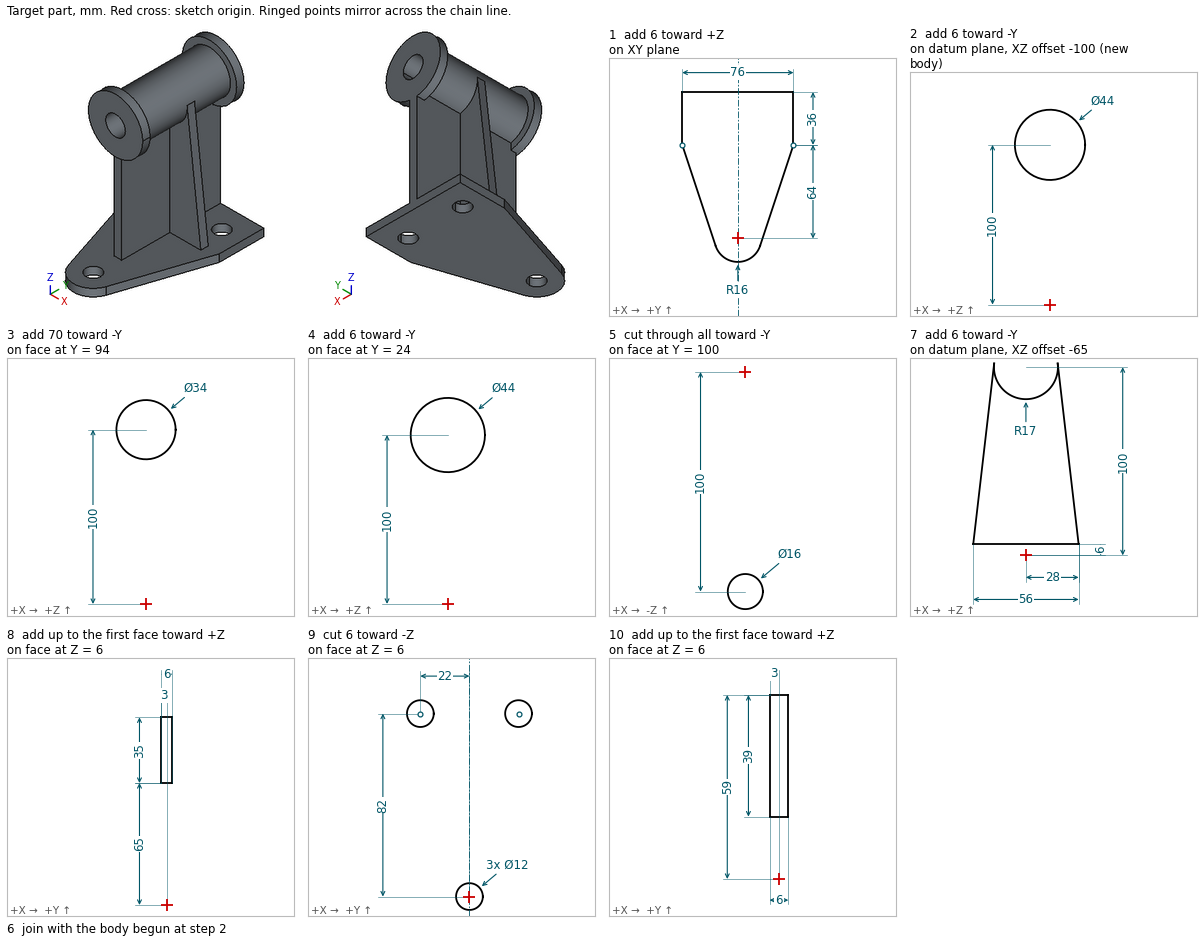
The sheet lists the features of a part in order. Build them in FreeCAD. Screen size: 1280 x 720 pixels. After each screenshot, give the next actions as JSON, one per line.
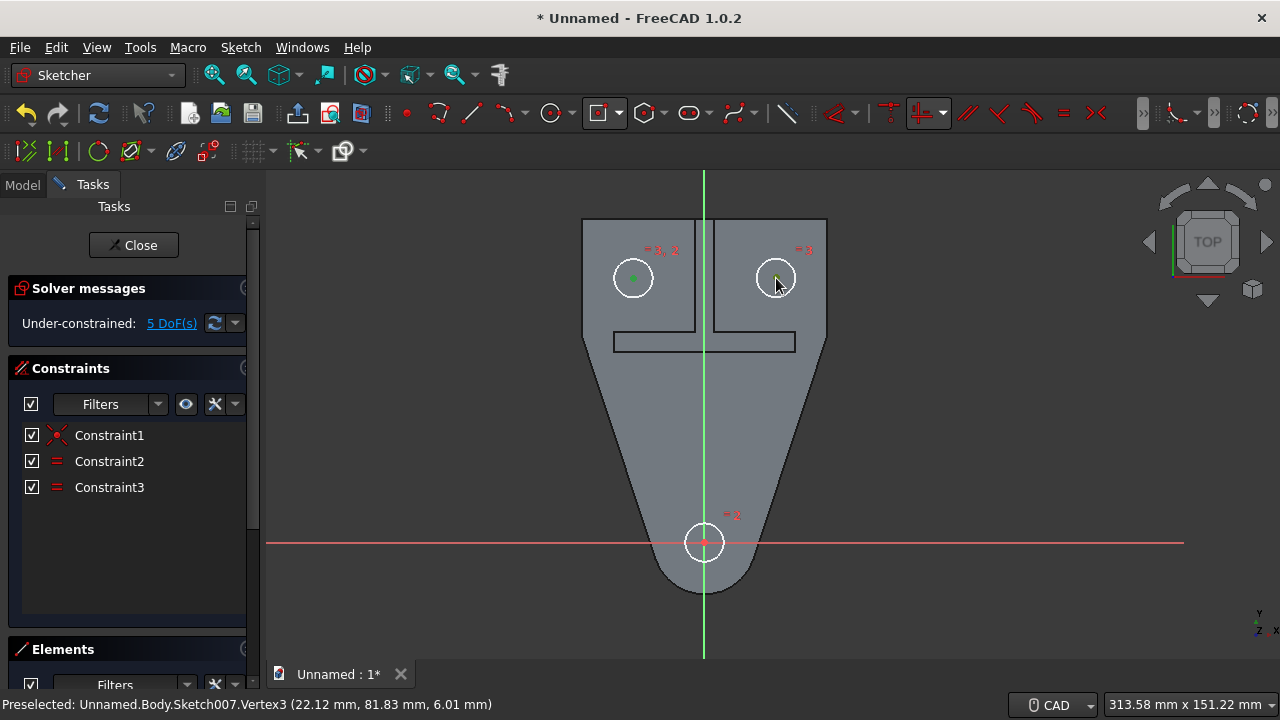
{"action": "left_click", "coordinate": [704, 600]}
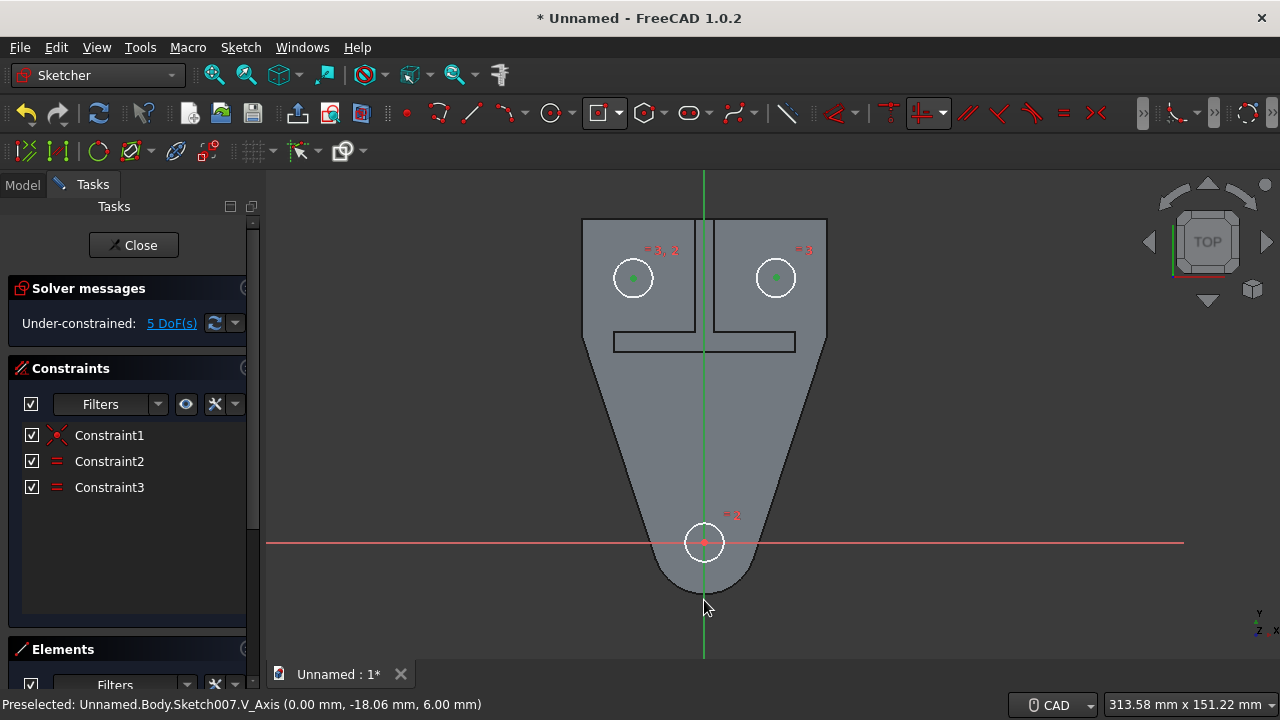
{"action": "key", "text": "s"}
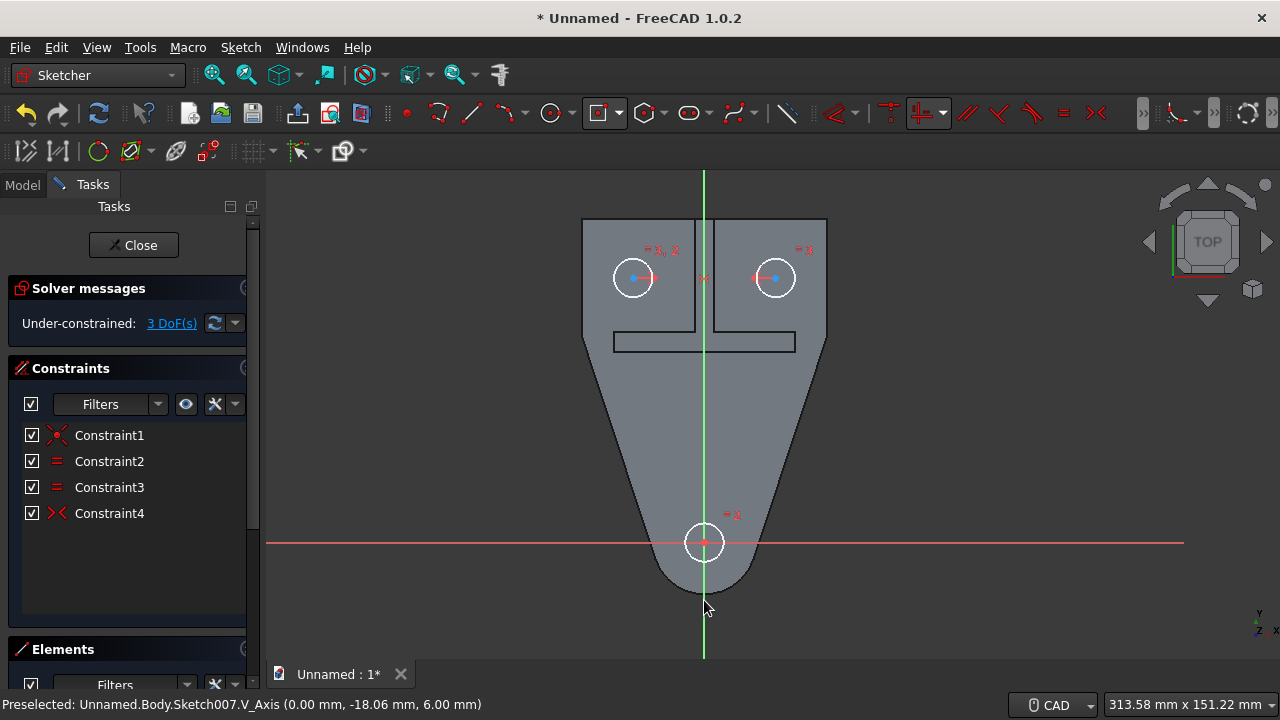
{"action": "left_click", "coordinate": [834, 114]}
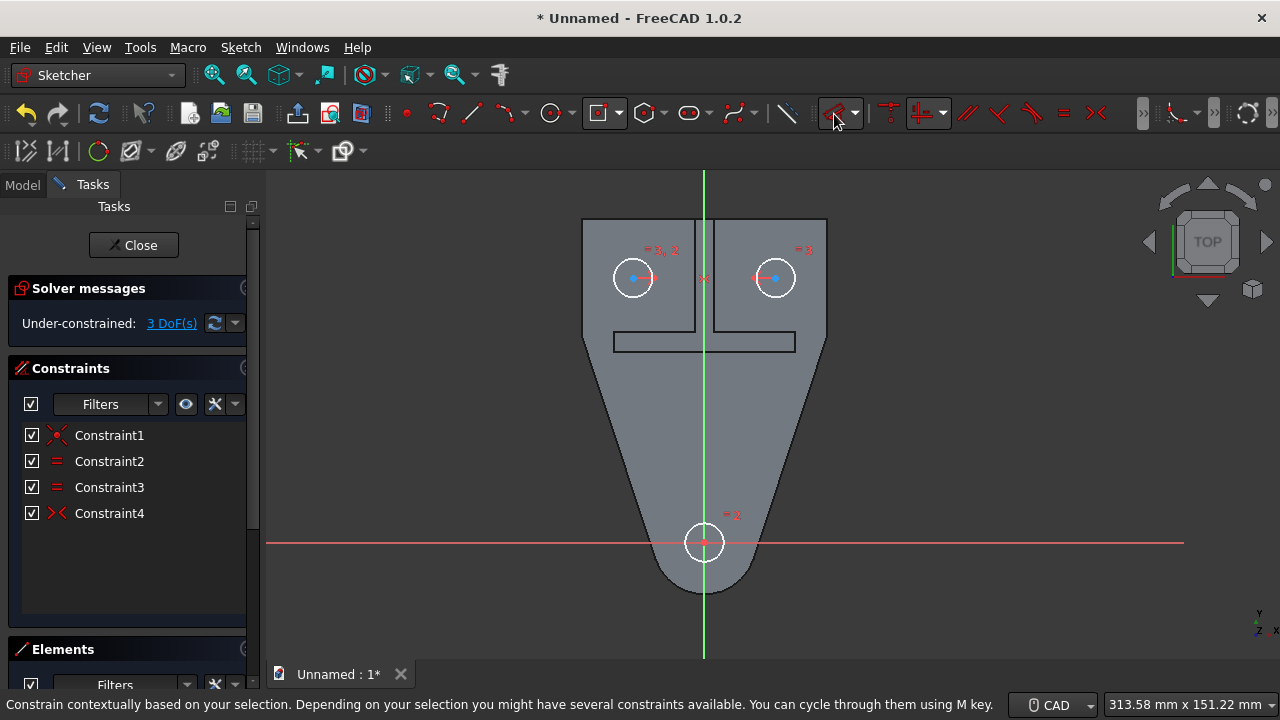
{"action": "left_click", "coordinate": [718, 529]}
{"action": "left_click", "coordinate": [741, 506]}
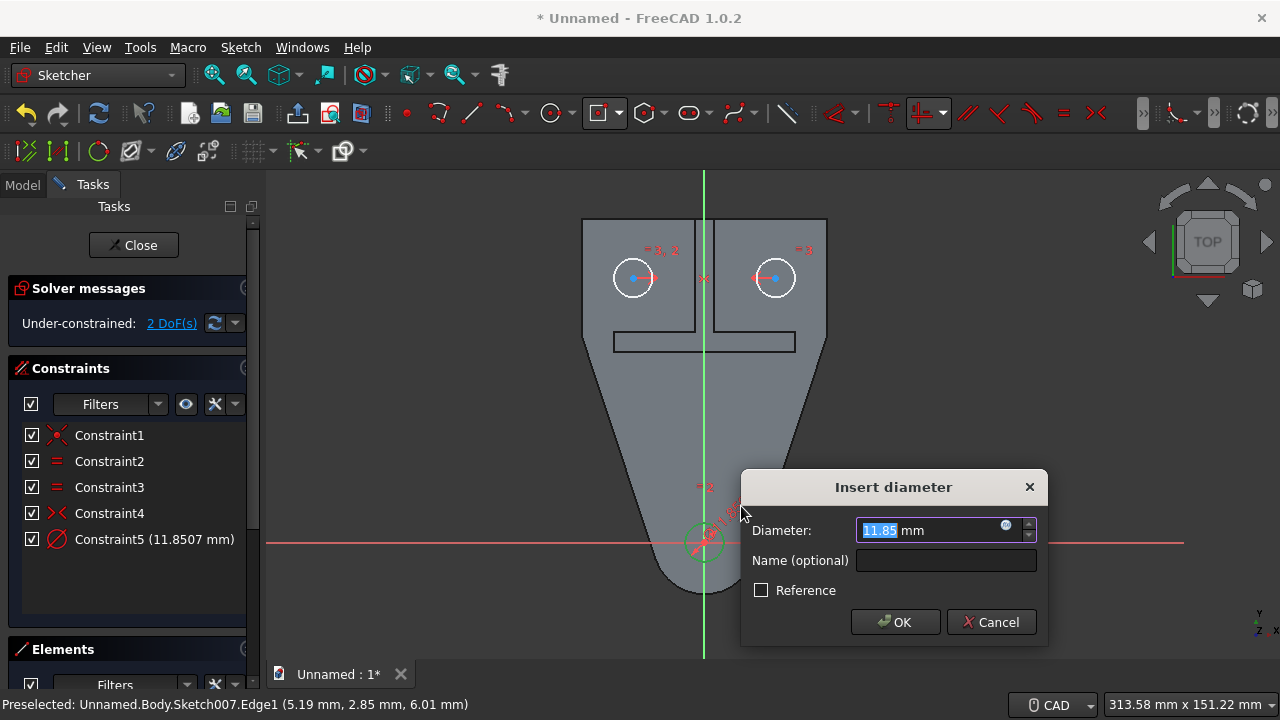
{"action": "type", "text": "12"}
{"action": "key", "text": "Return"}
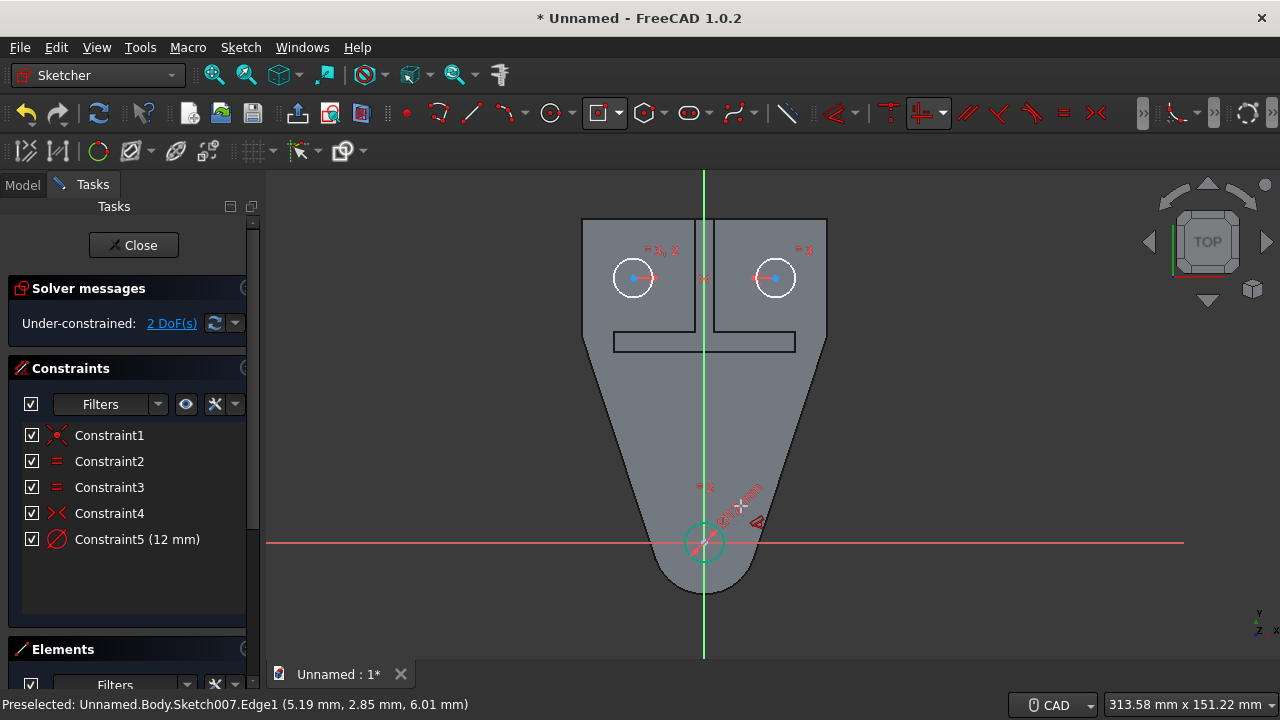
{"action": "left_click", "coordinate": [633, 278]}
{"action": "left_click", "coordinate": [669, 577]}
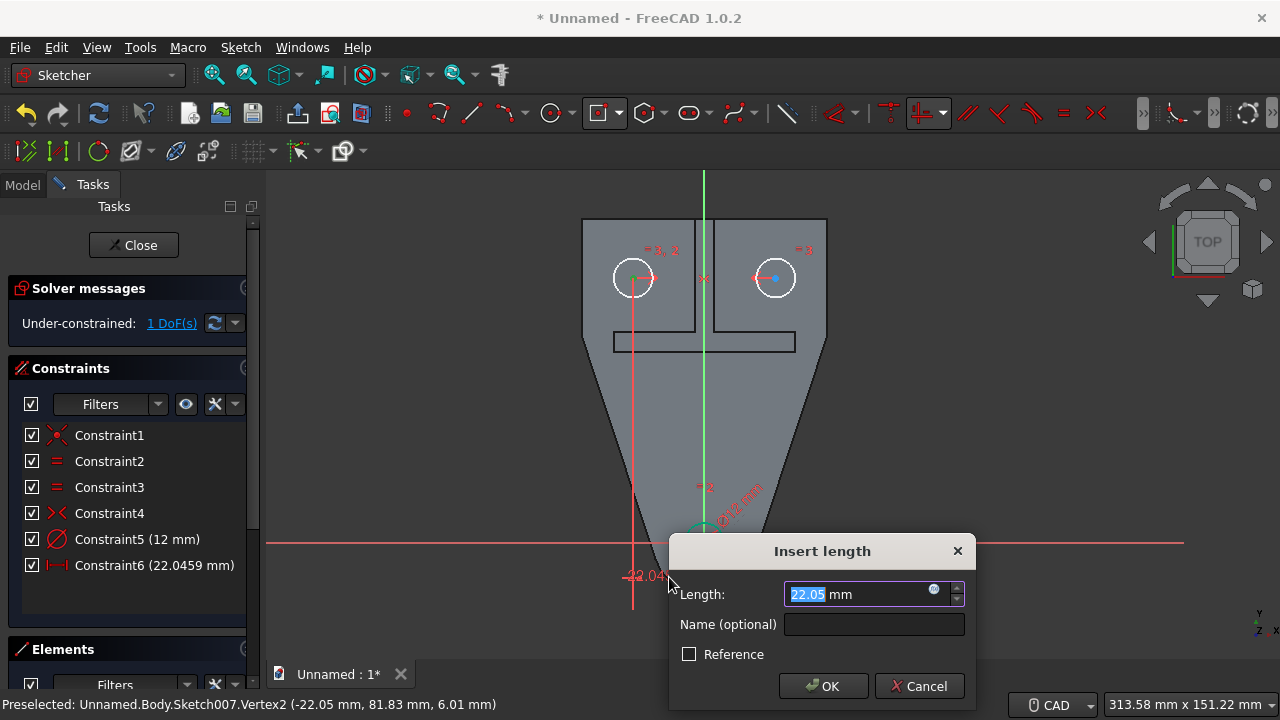
{"action": "type", "text": "22"}
{"action": "key", "text": "Return"}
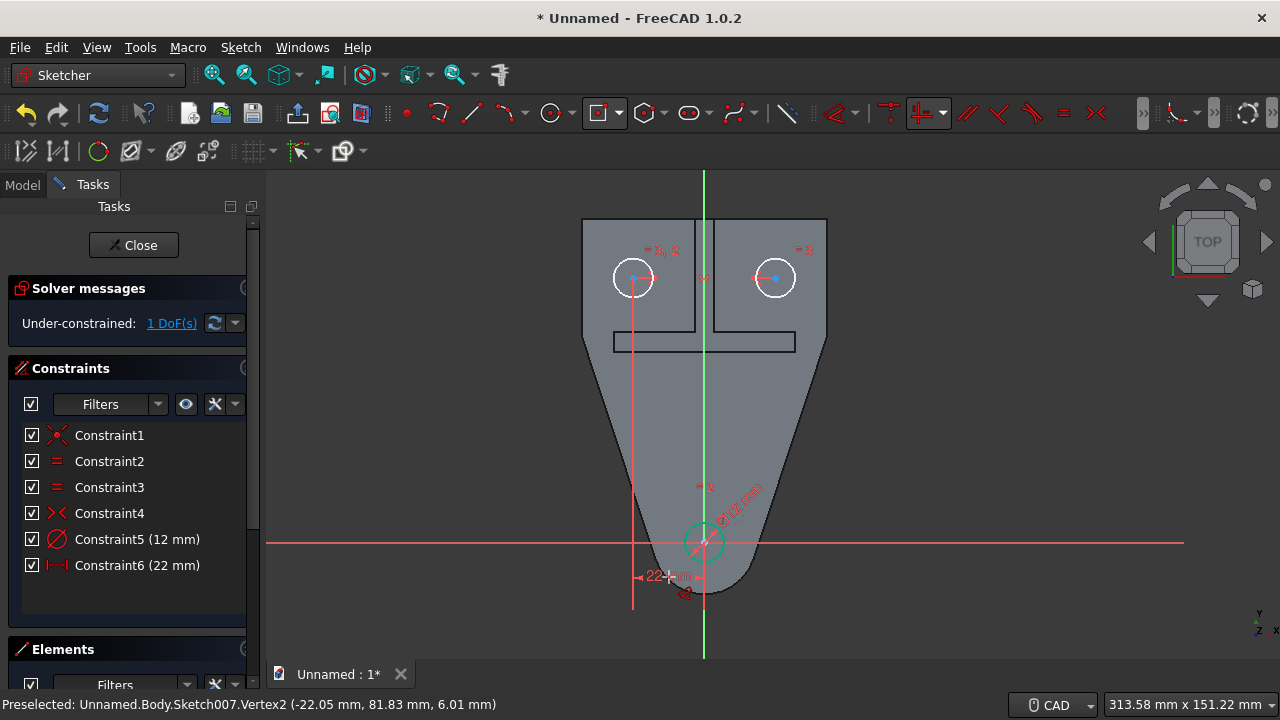
{"action": "left_click", "coordinate": [633, 278]}
{"action": "left_click", "coordinate": [599, 410]}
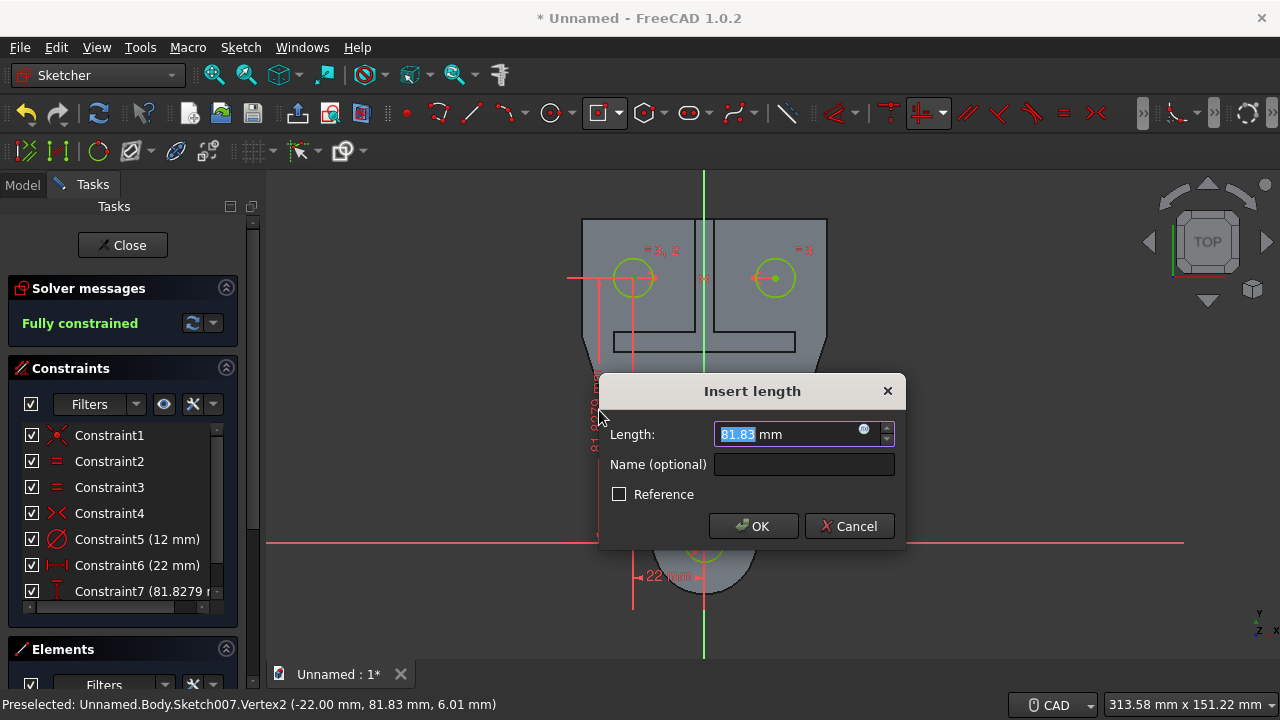
{"action": "type", "text": "82"}
{"action": "key", "text": "Return"}
{"action": "key", "text": "Escape"}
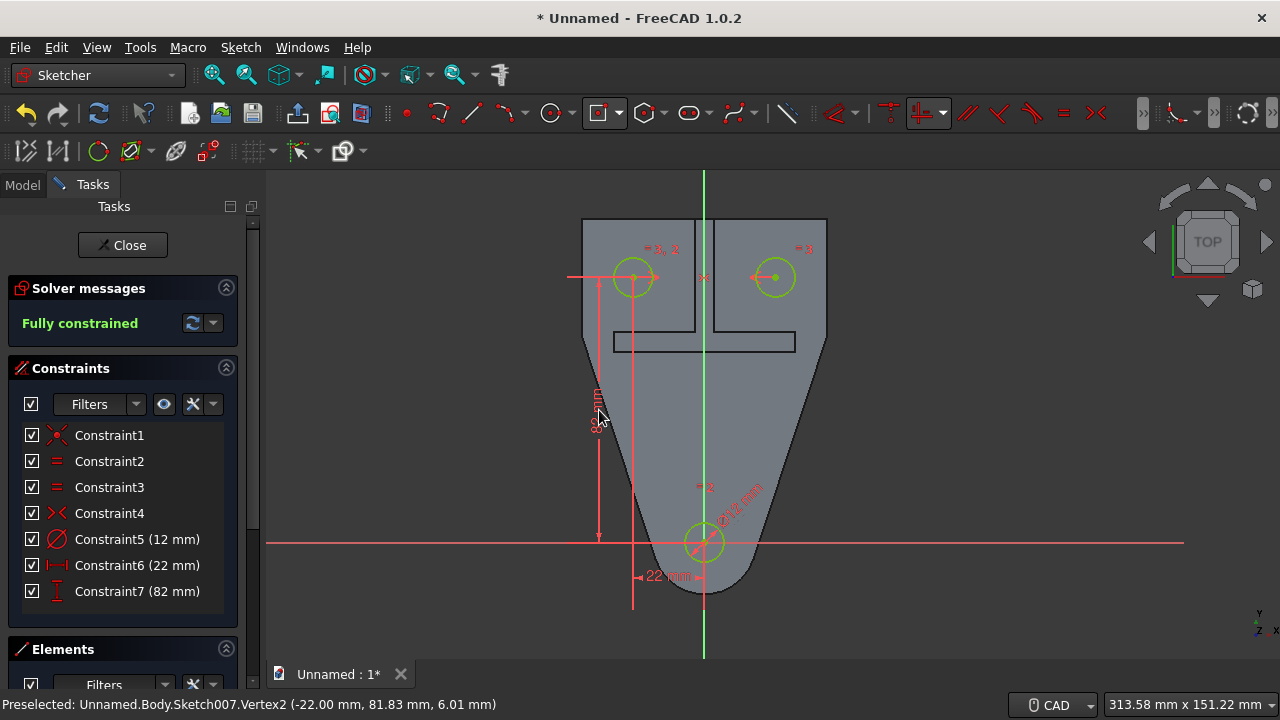
{"action": "left_click", "coordinate": [123, 245]}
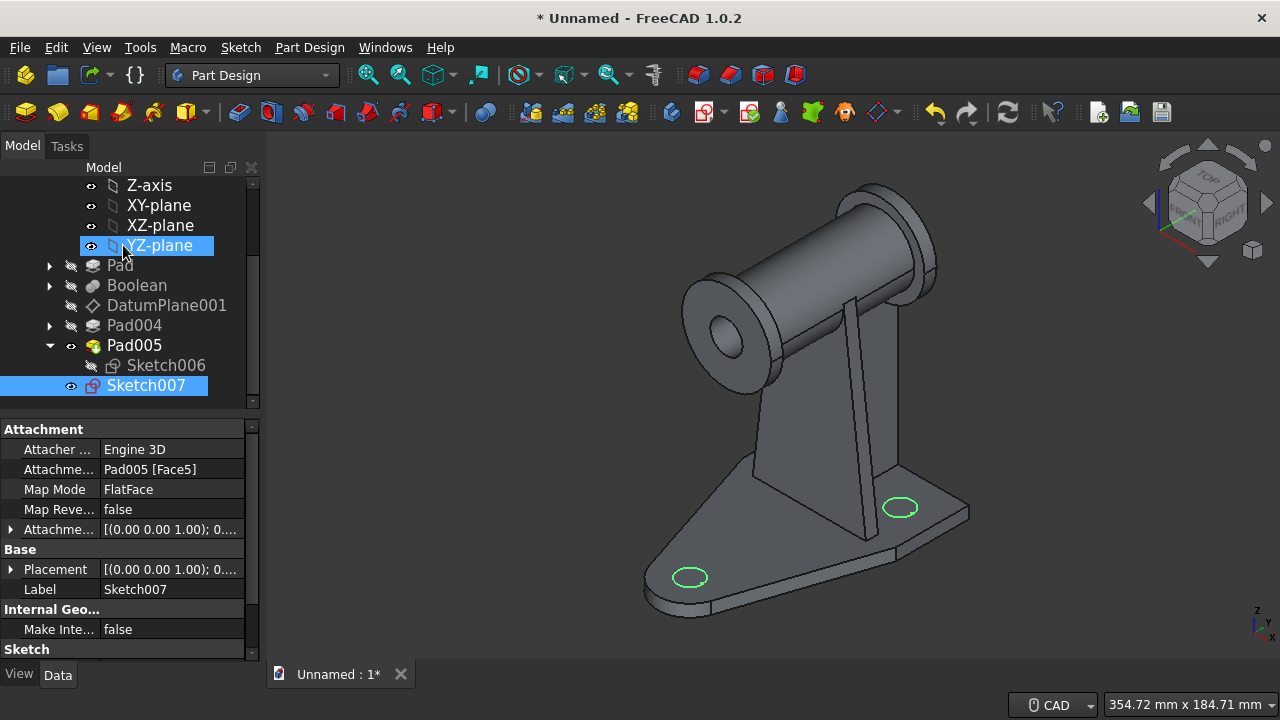
{"action": "left_click", "coordinate": [240, 112]}